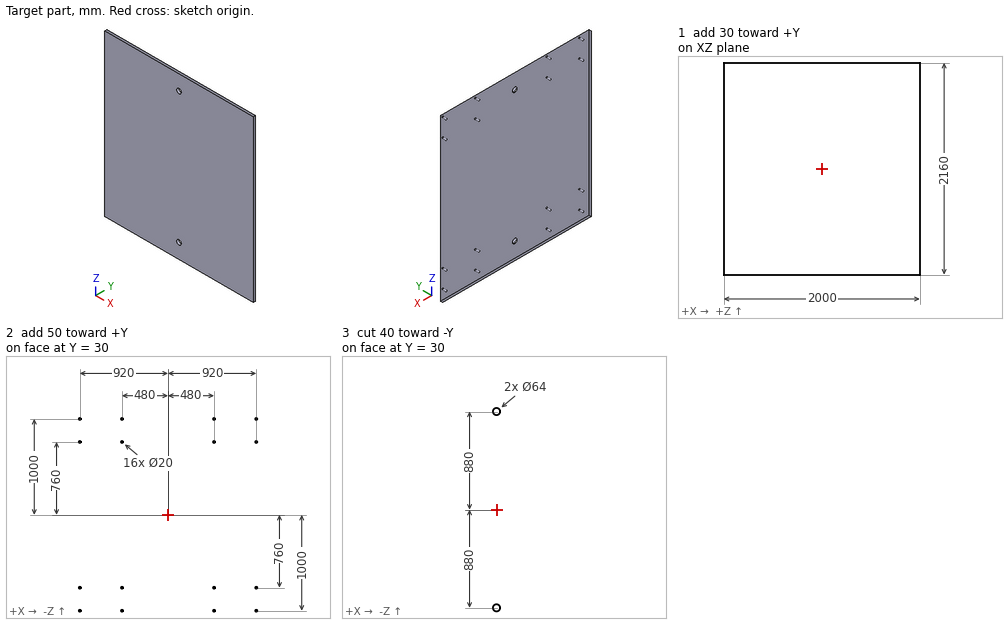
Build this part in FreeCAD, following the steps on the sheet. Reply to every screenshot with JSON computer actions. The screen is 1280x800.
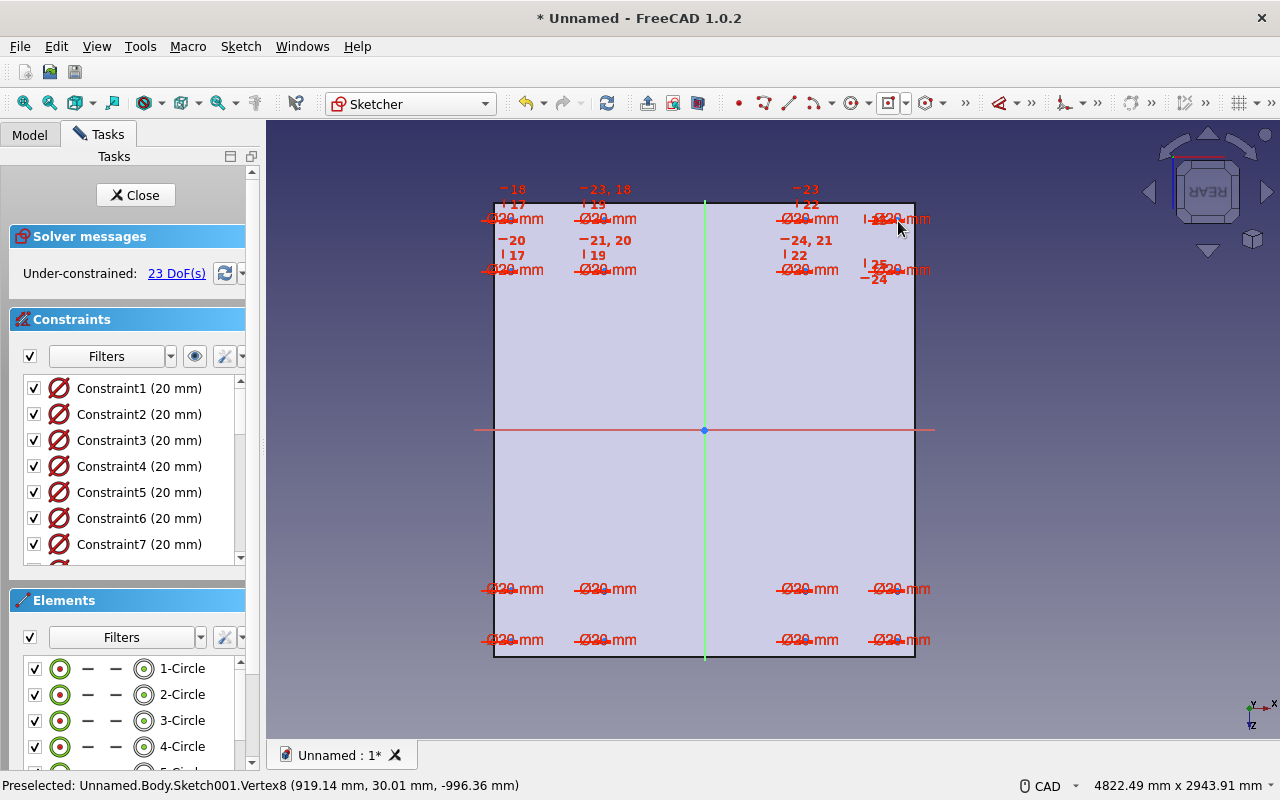
{"action": "left_click", "coordinate": [806, 221]}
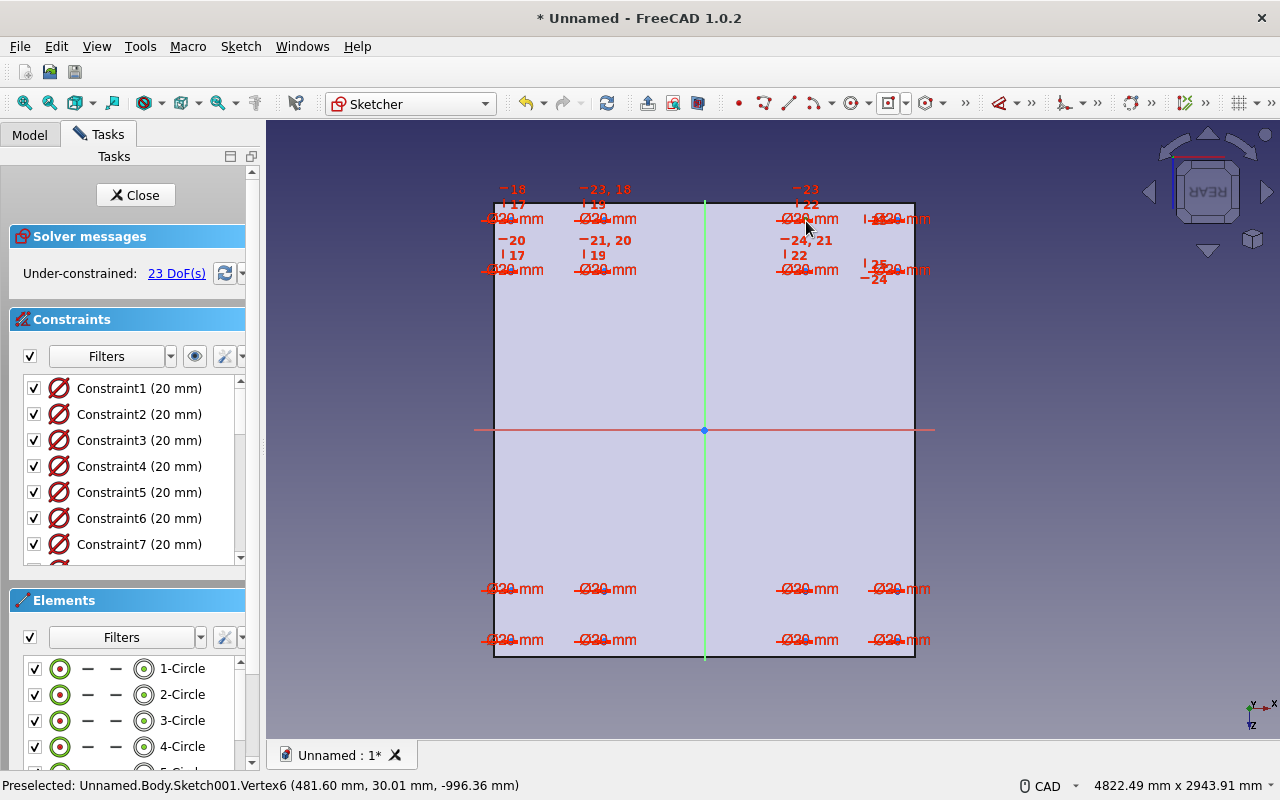
{"action": "left_click", "coordinate": [898, 221]}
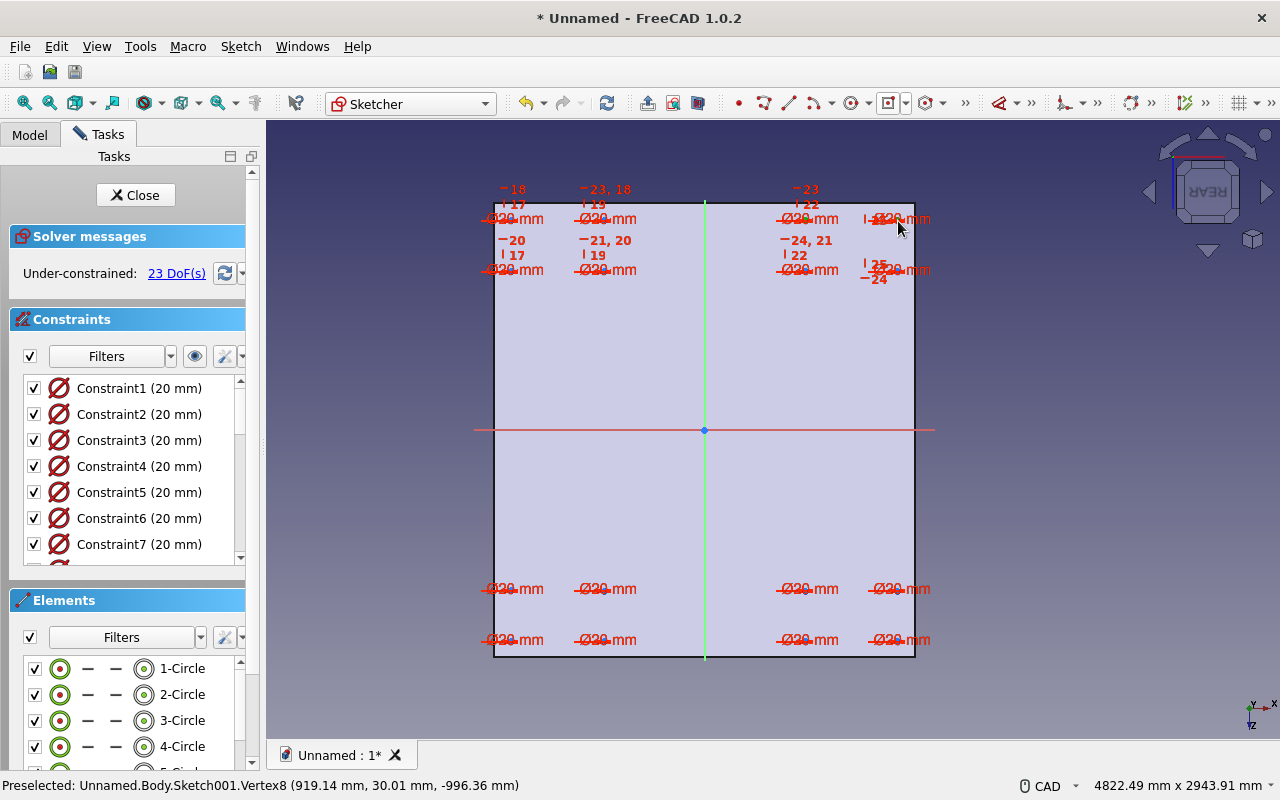
{"action": "key", "text": "h"}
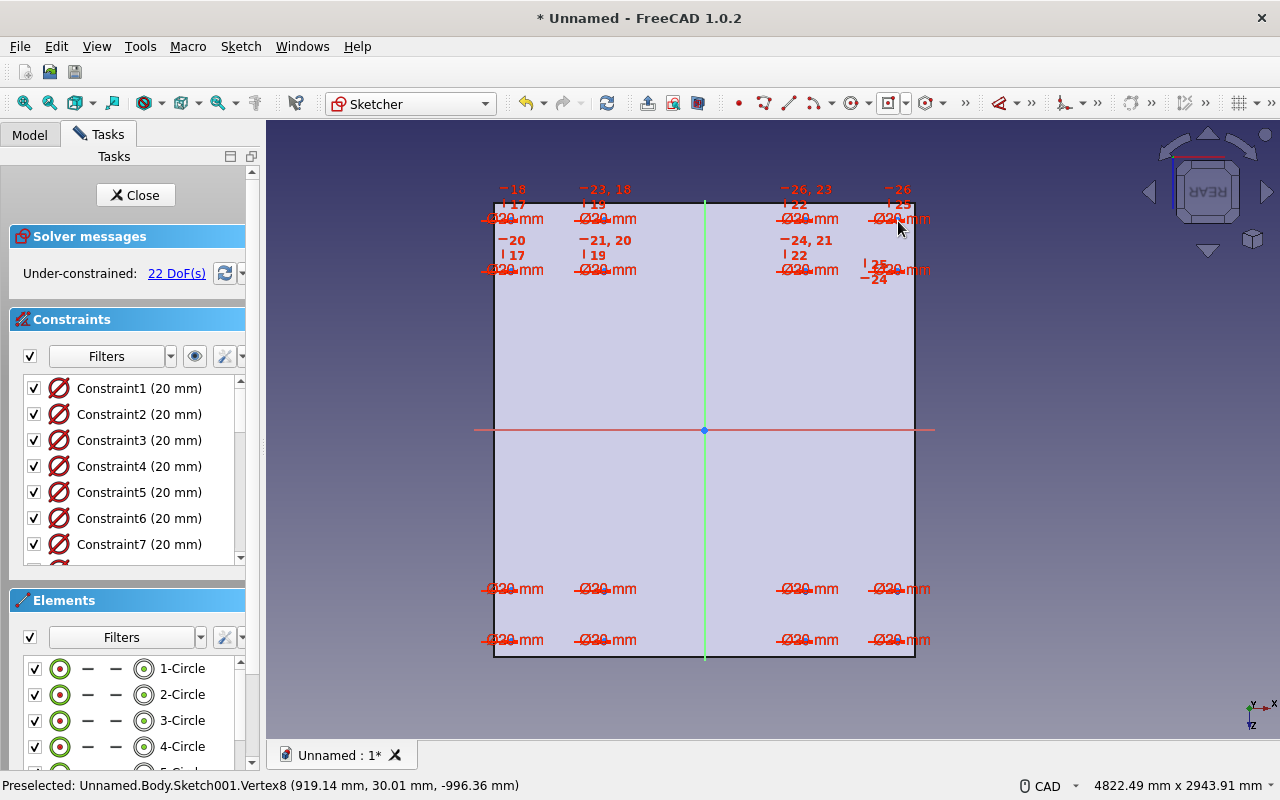
{"action": "left_click", "coordinate": [898, 272]}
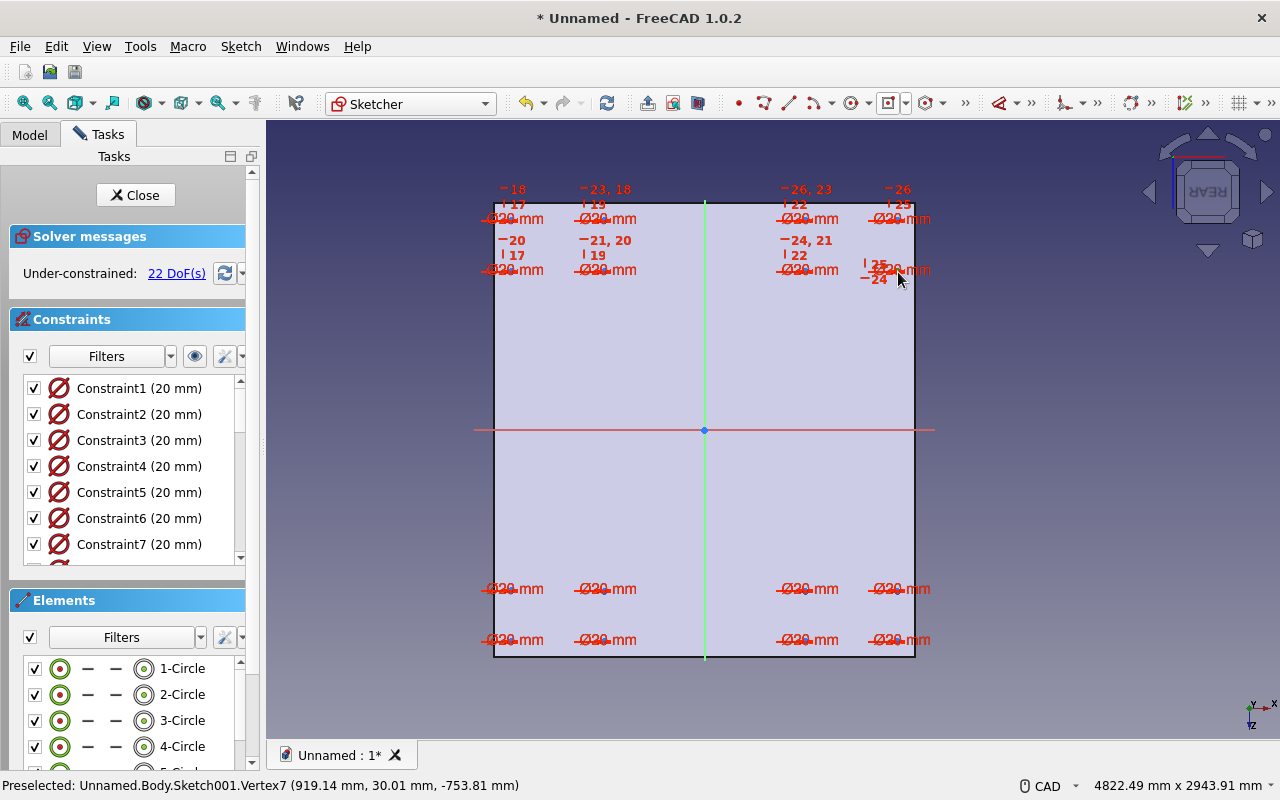
{"action": "left_click", "coordinate": [898, 642]}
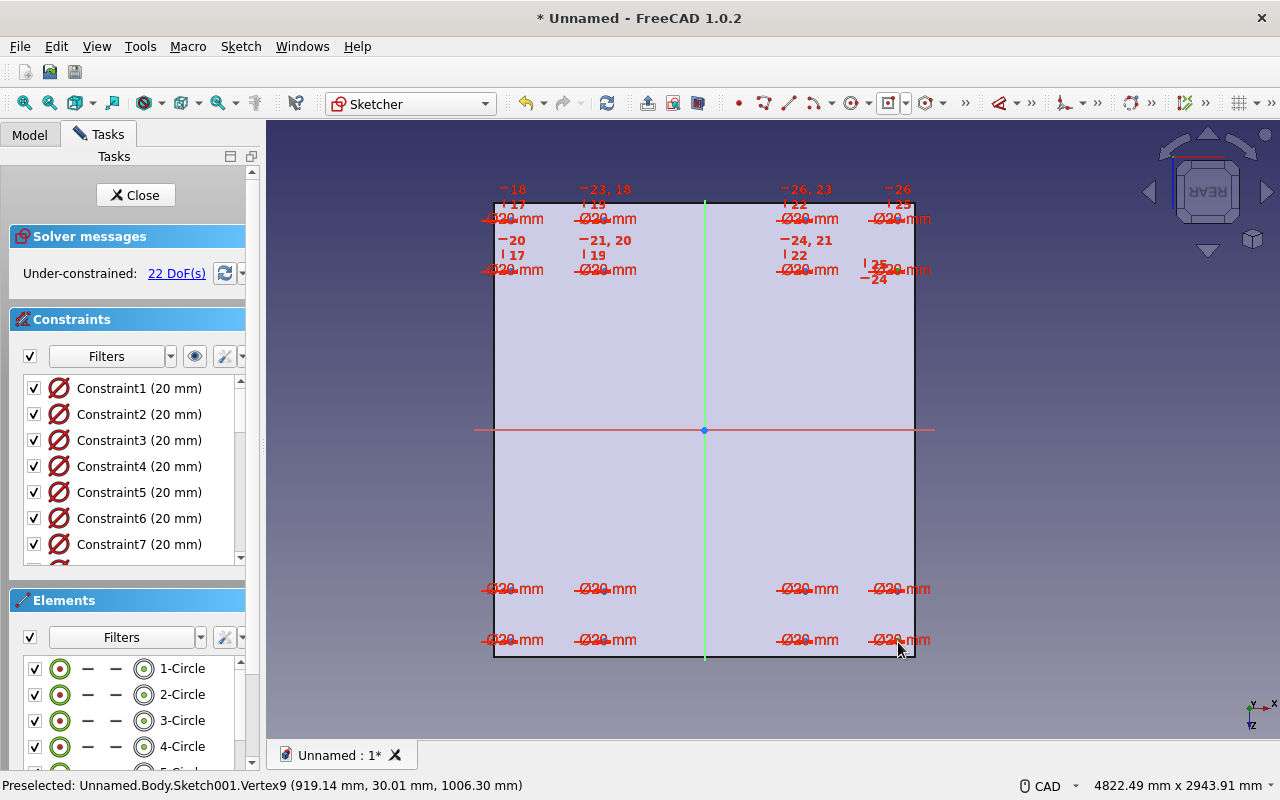
{"action": "key", "text": "v"}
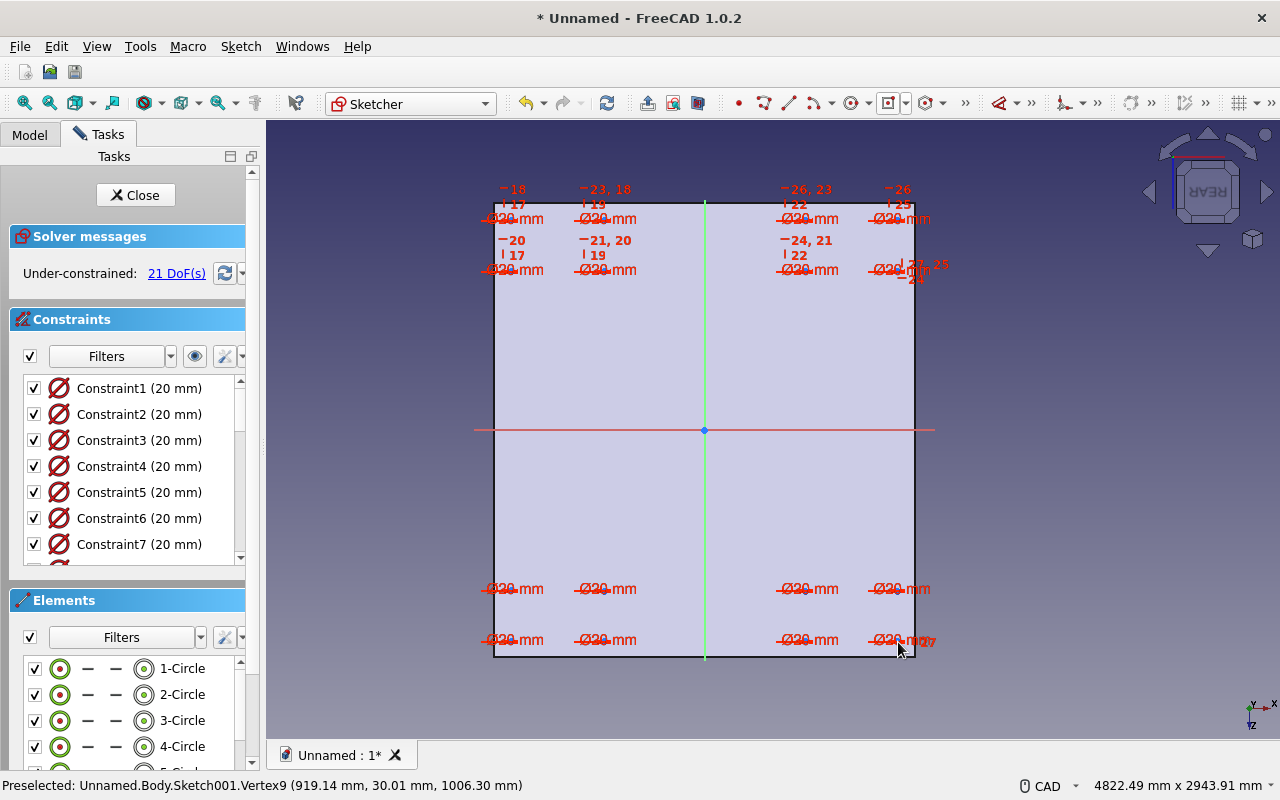
{"action": "left_click", "coordinate": [898, 642]}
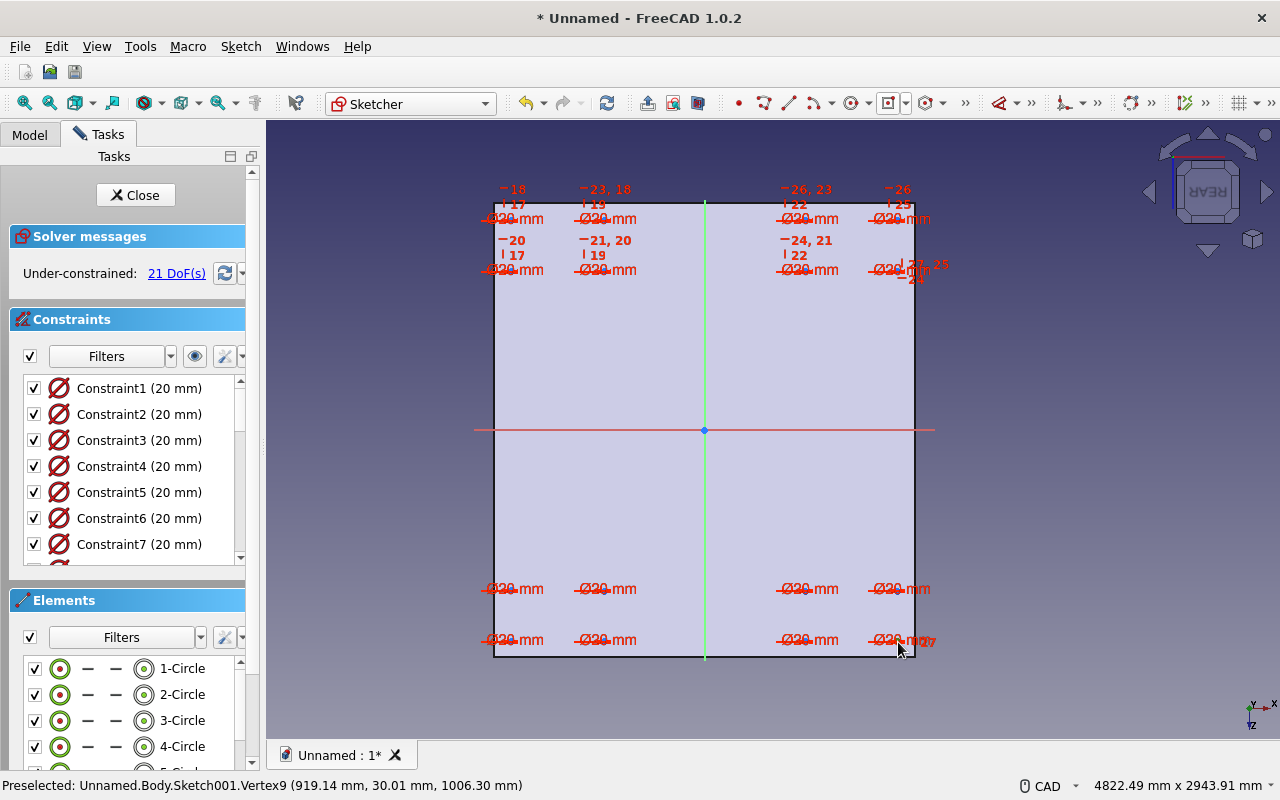
{"action": "left_click", "coordinate": [898, 591]}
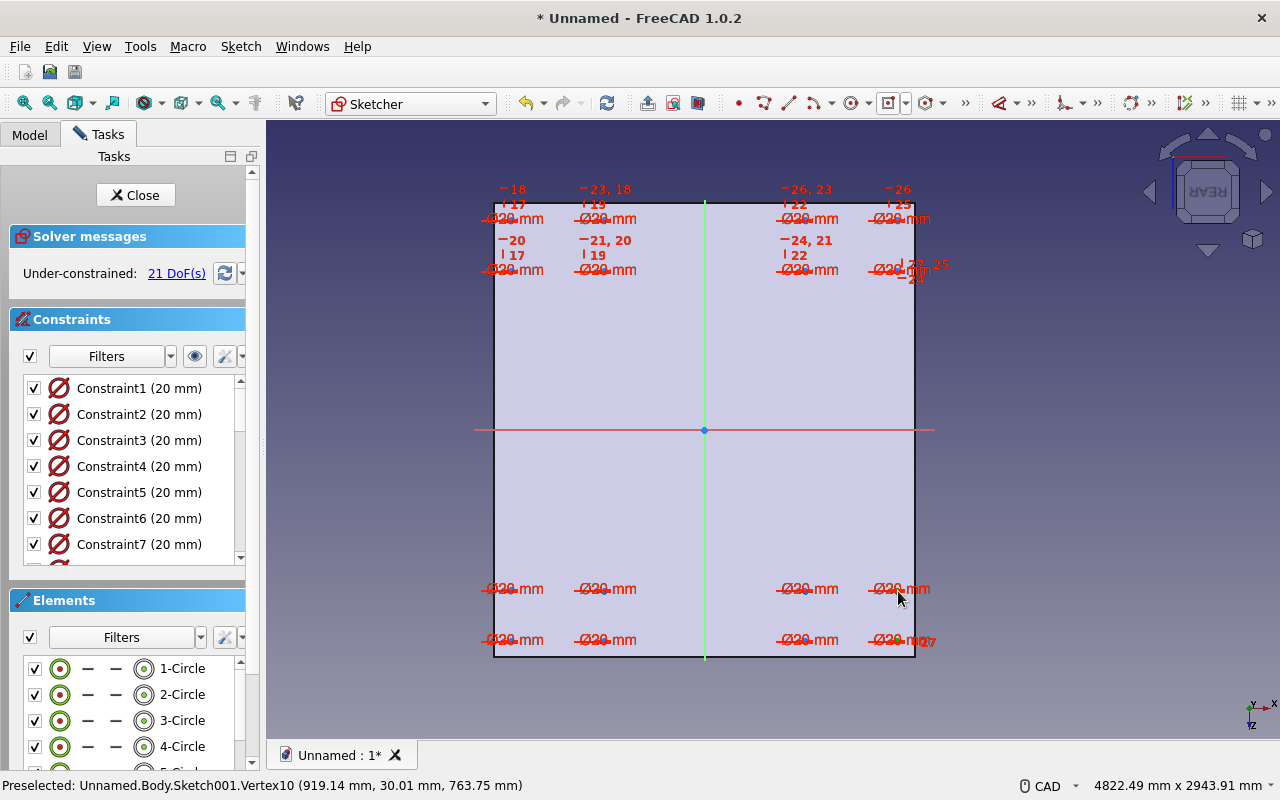
{"action": "key", "text": "v"}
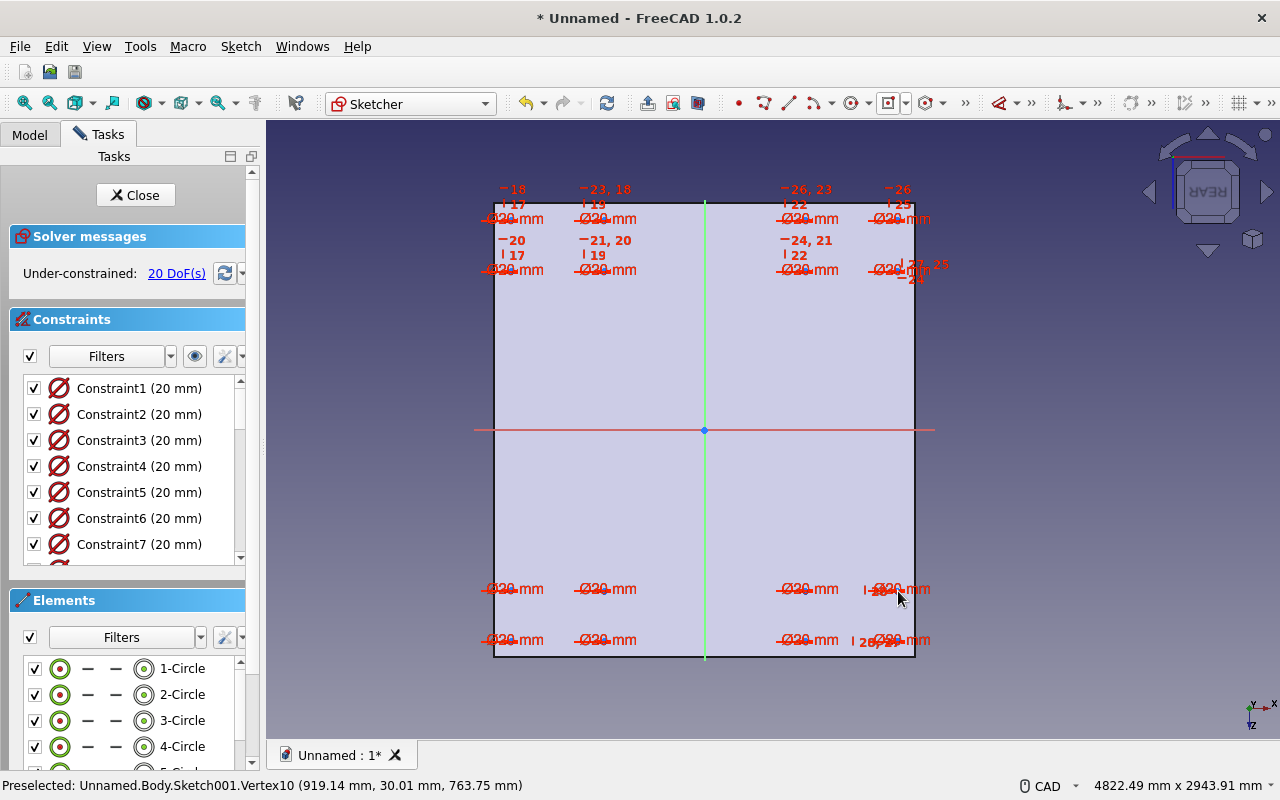
{"action": "left_click", "coordinate": [806, 272]}